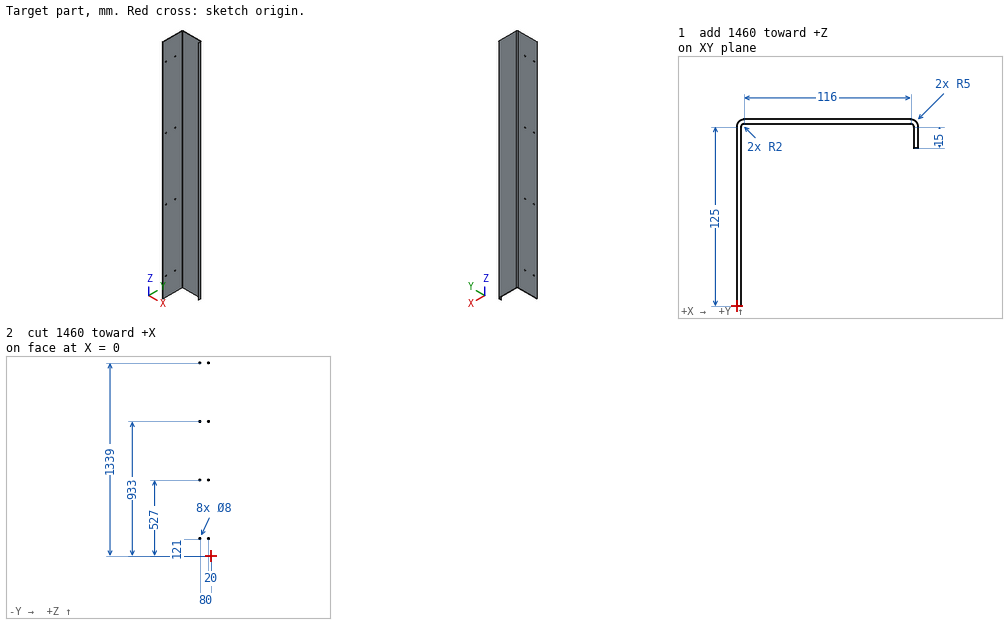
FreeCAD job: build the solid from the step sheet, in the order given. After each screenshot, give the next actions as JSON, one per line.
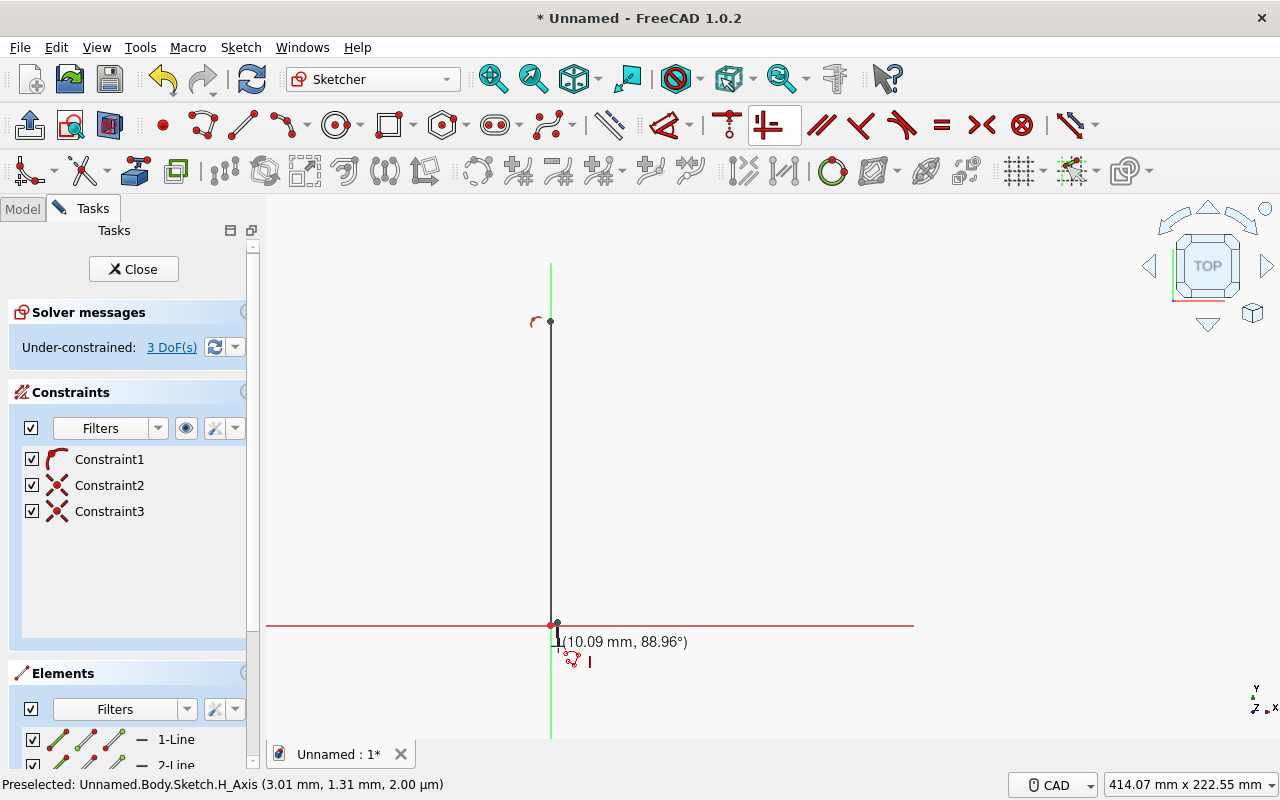
{"action": "scroll", "coordinate": [558, 320], "scroll_direction": "up", "scroll_amount": 4}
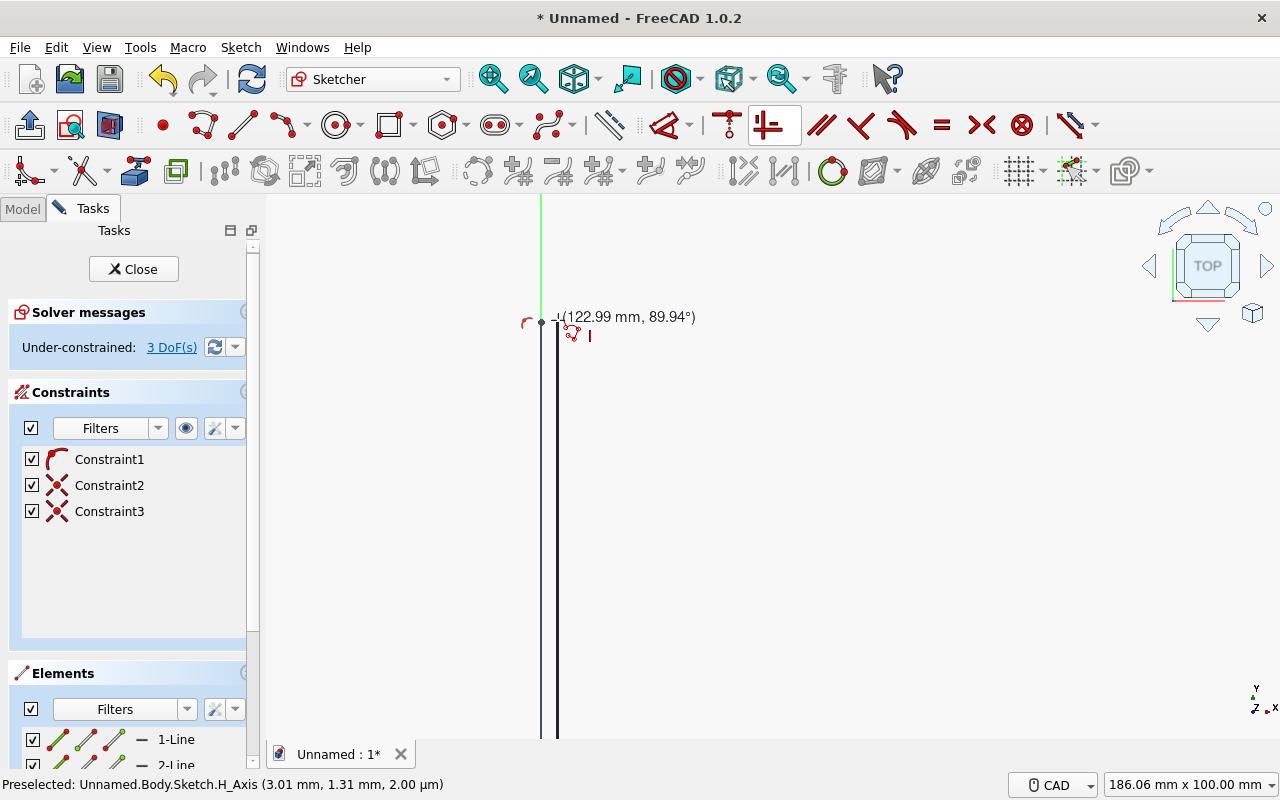
{"action": "left_click", "coordinate": [557, 319]}
{"action": "right_click", "coordinate": [557, 319]}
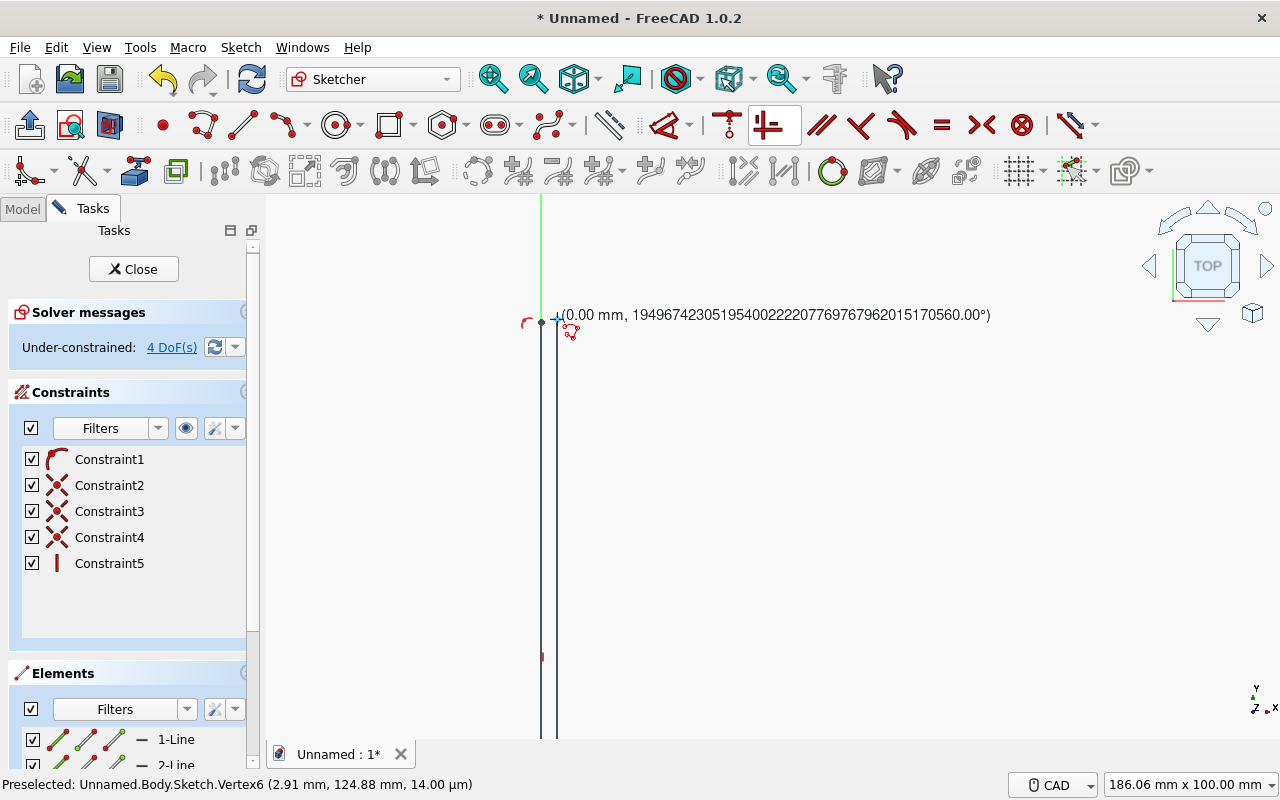
{"action": "key", "text": "g l"}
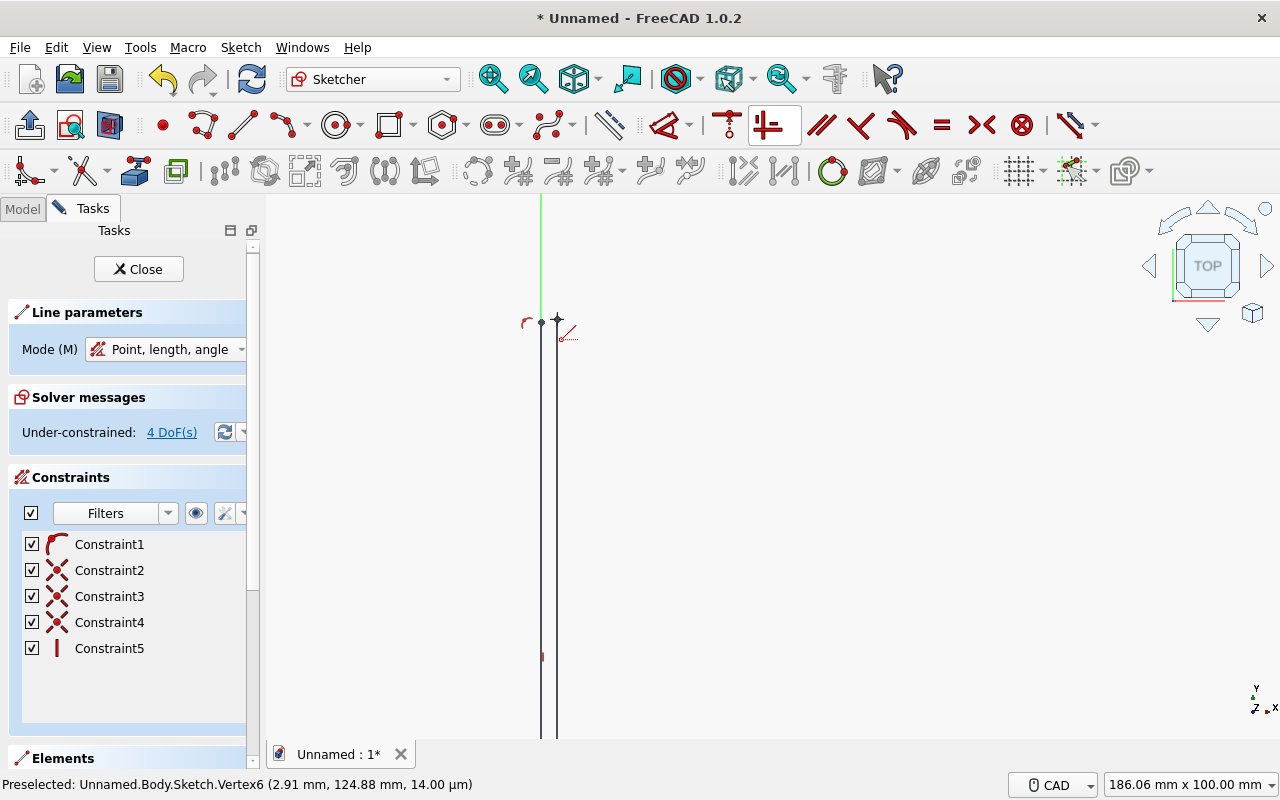
{"action": "left_click", "coordinate": [568, 308]}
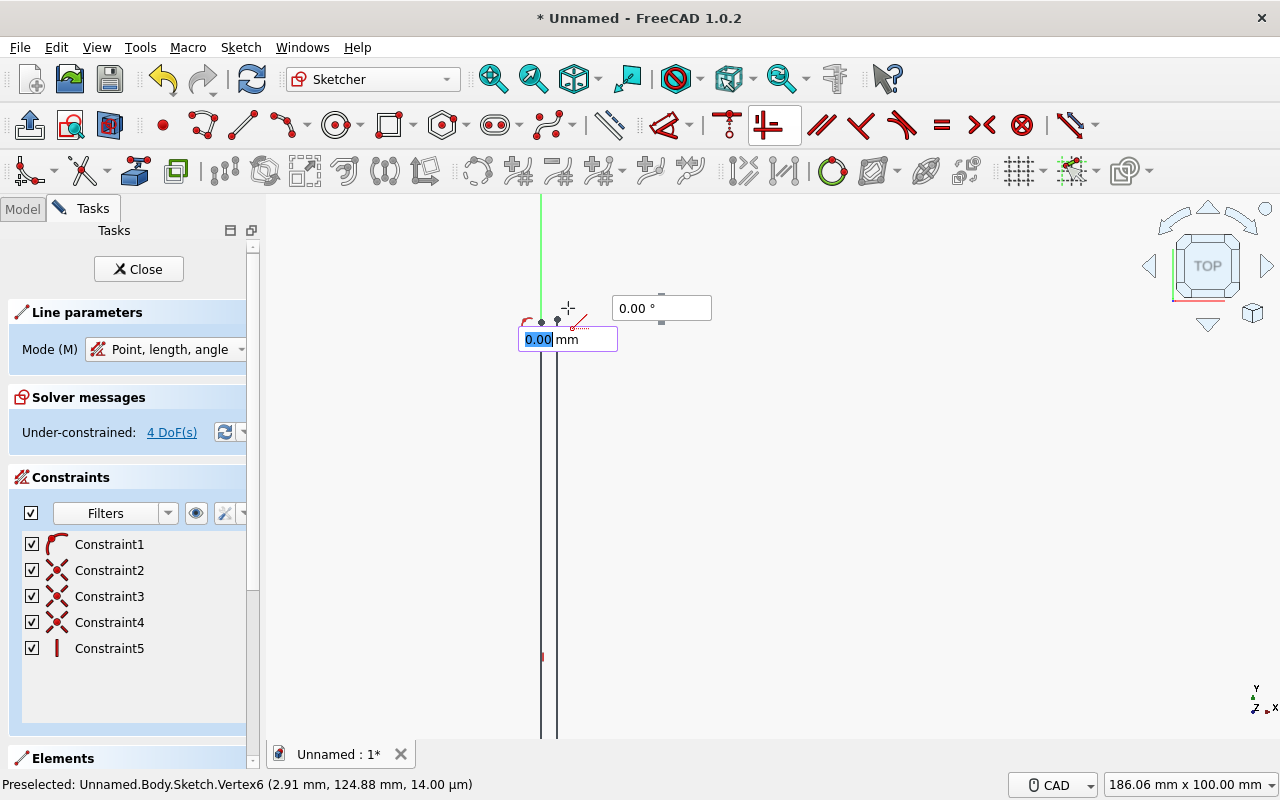
{"action": "scroll", "coordinate": [558, 320], "scroll_direction": "down", "scroll_amount": 4}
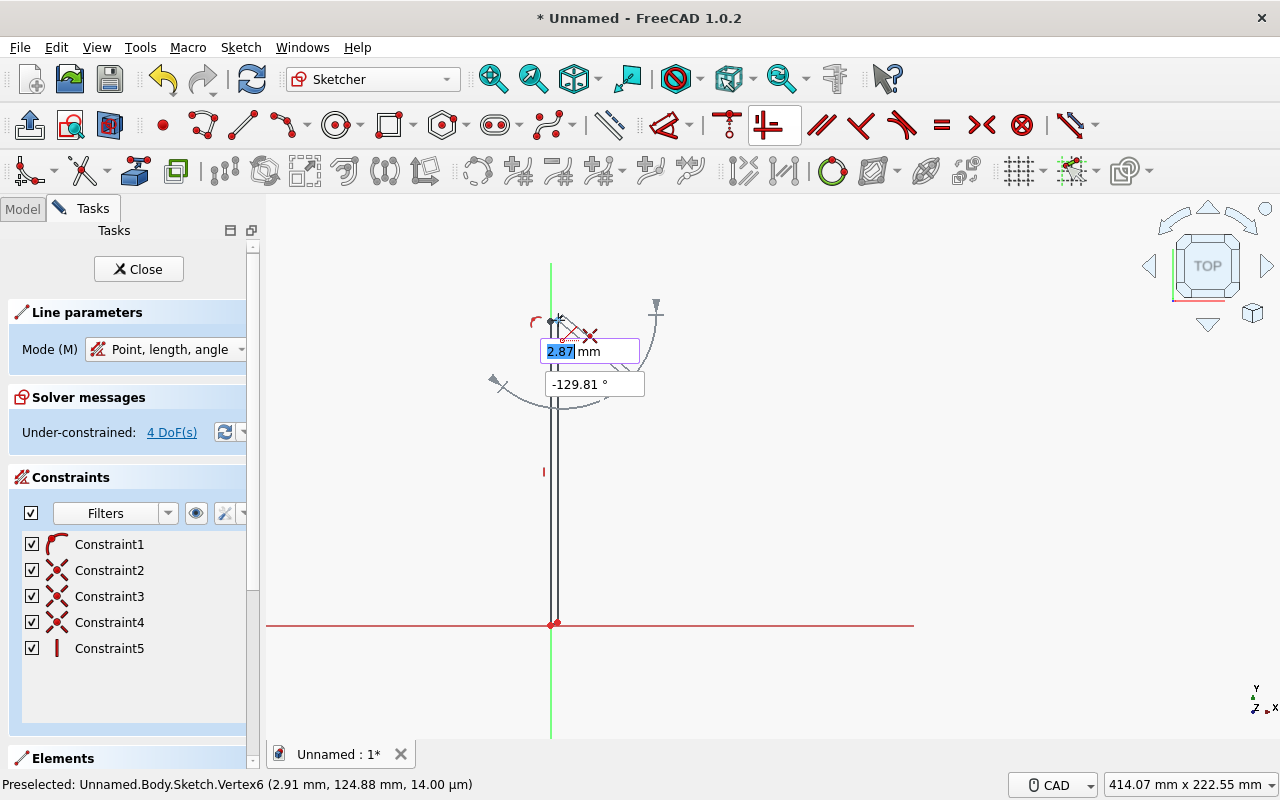
{"action": "left_click", "coordinate": [847, 315]}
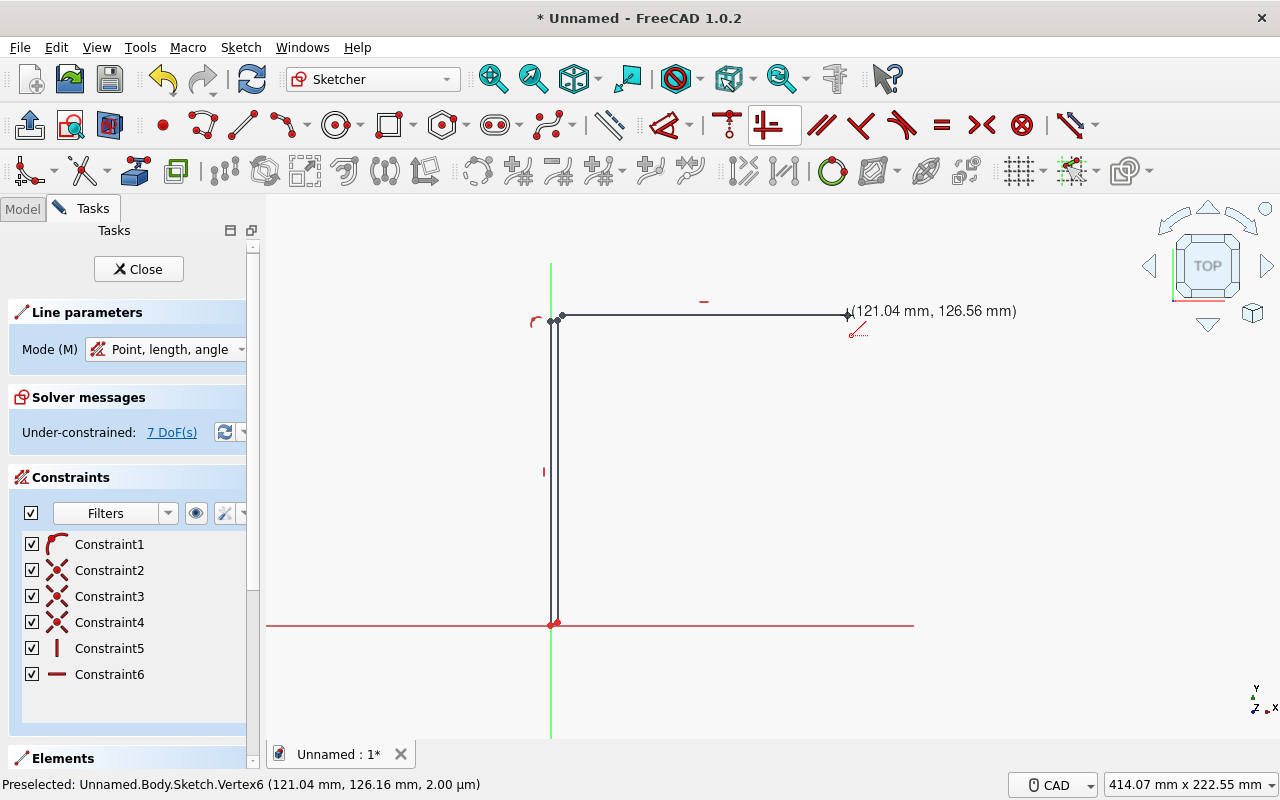
{"action": "key", "text": "g m"}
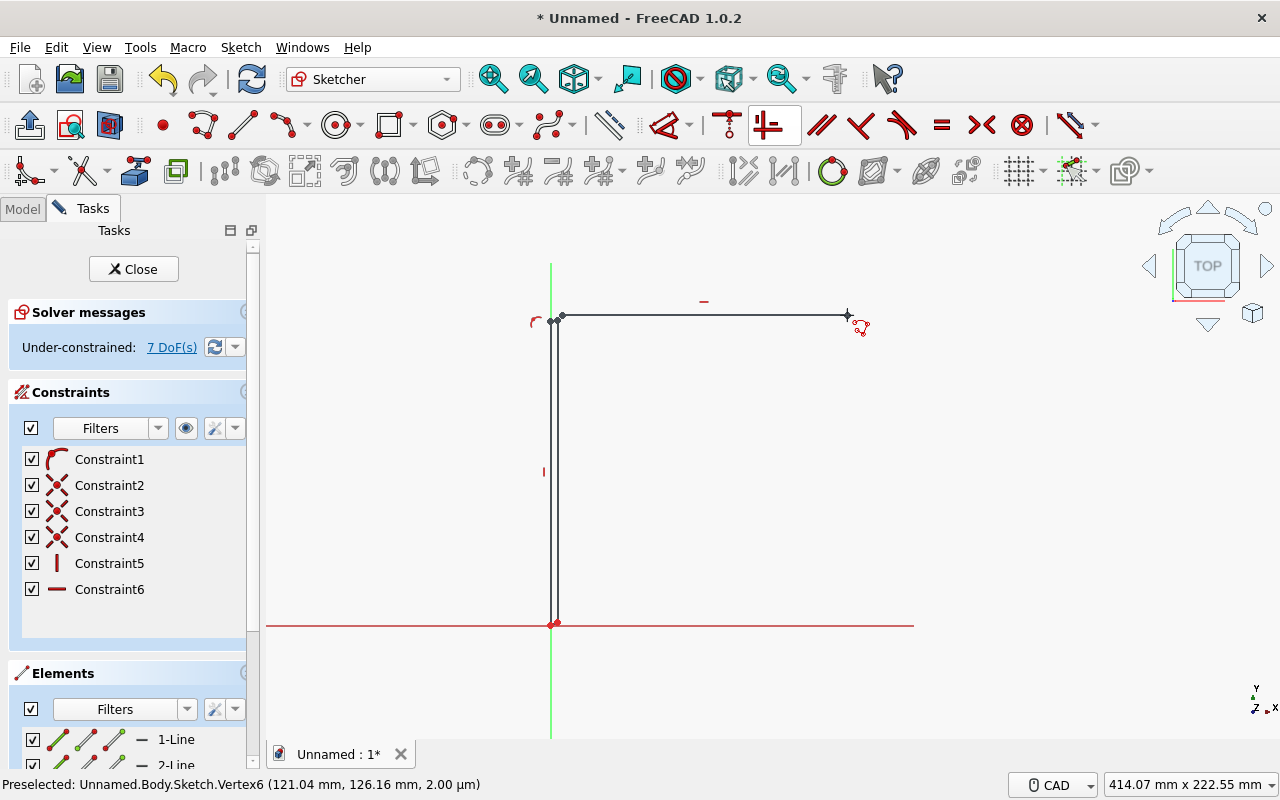
{"action": "scroll", "coordinate": [852, 320], "scroll_direction": "up", "scroll_amount": 5}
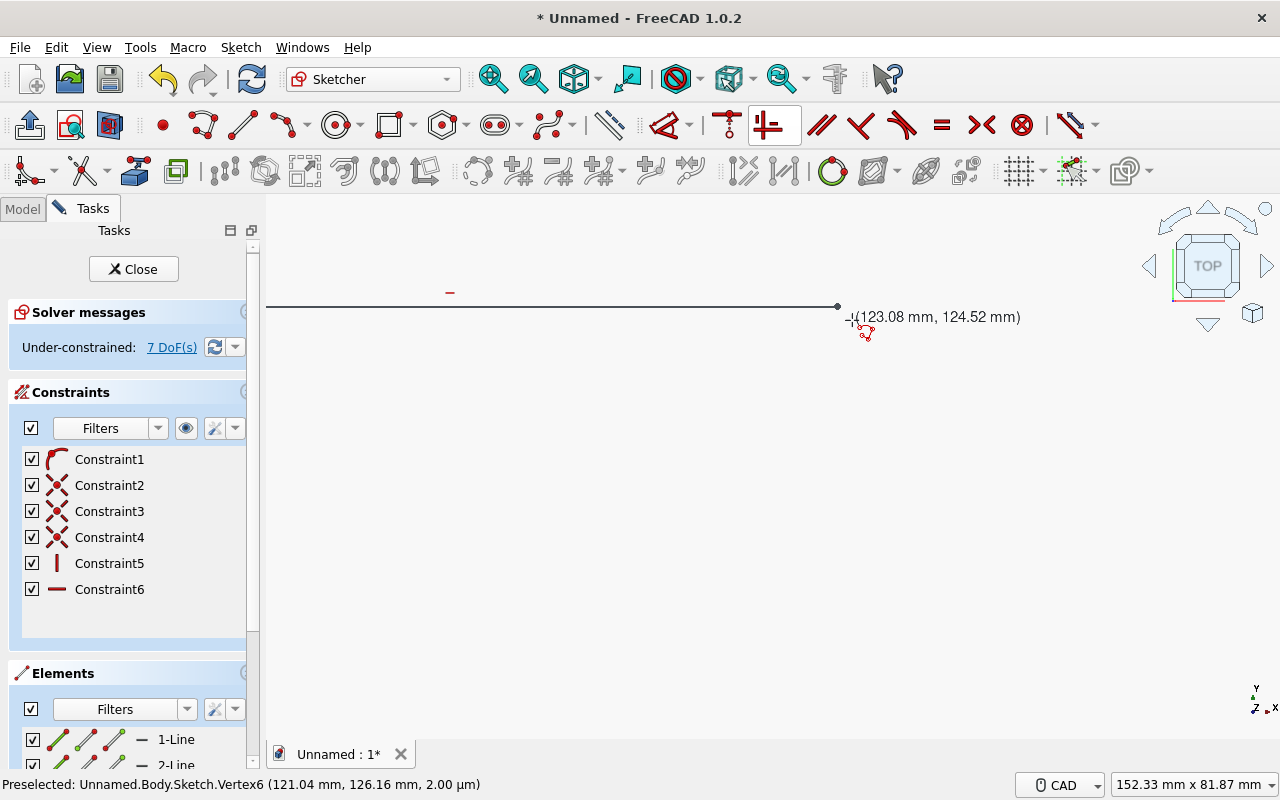
{"action": "left_click", "coordinate": [850, 319]}
{"action": "left_click", "coordinate": [850, 419]}
{"action": "left_click", "coordinate": [870, 419]}
{"action": "left_click", "coordinate": [870, 319]}
{"action": "right_click", "coordinate": [870, 319]}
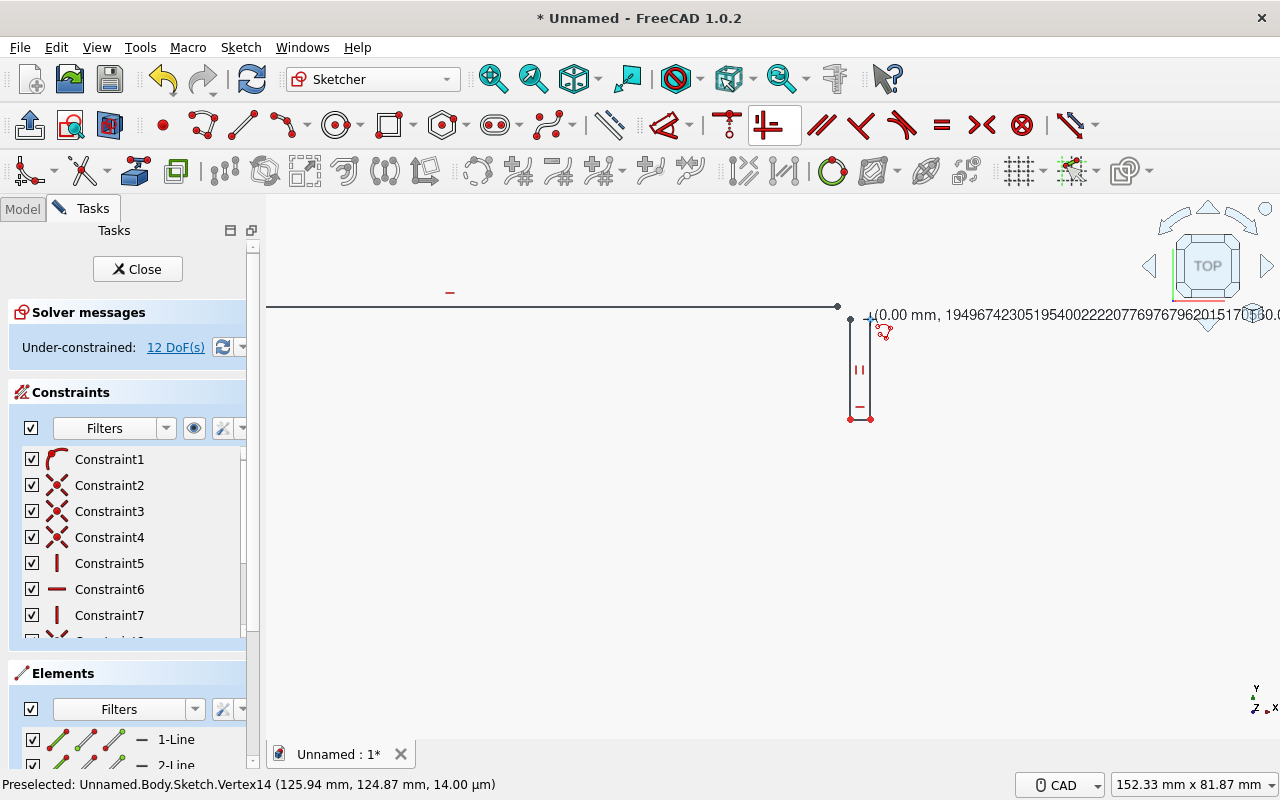
{"action": "left_click", "coordinate": [244, 126]}